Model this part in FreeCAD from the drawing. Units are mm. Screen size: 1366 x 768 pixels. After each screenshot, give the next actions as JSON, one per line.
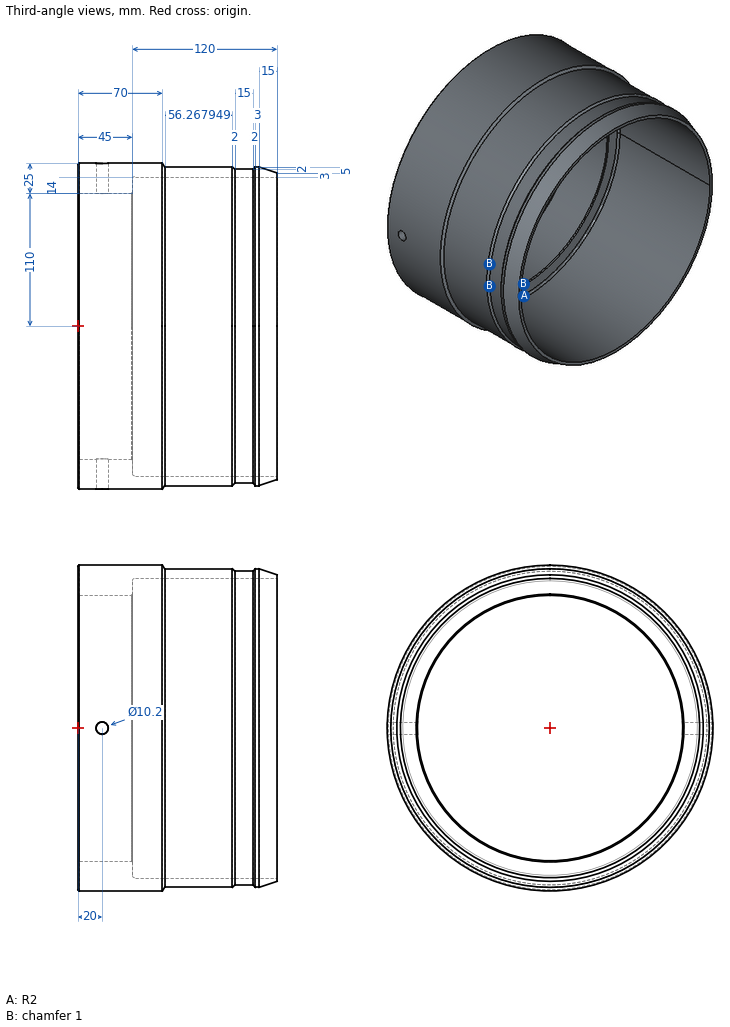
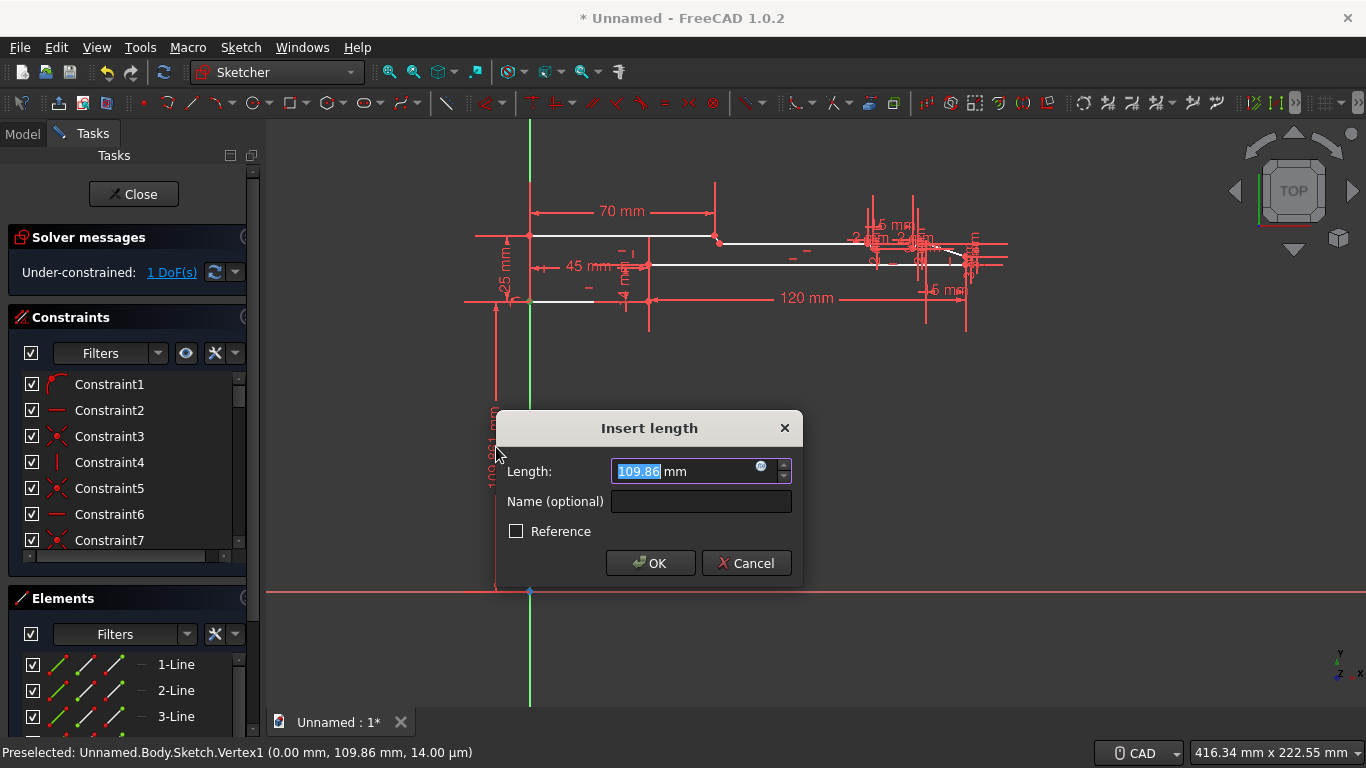
{"action": "type", "text": "110"}
{"action": "key", "text": "Return"}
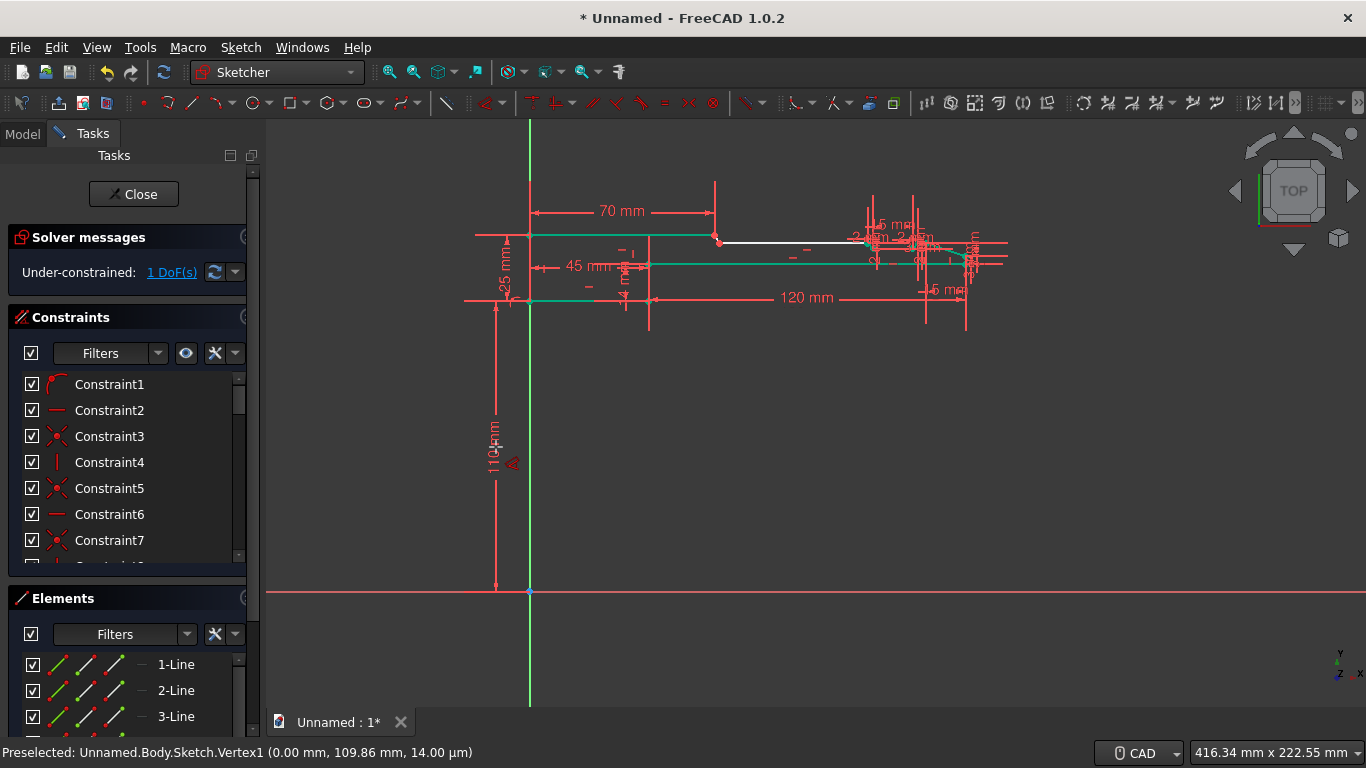
{"action": "left_click", "coordinate": [823, 243]}
{"action": "left_click", "coordinate": [794, 209]}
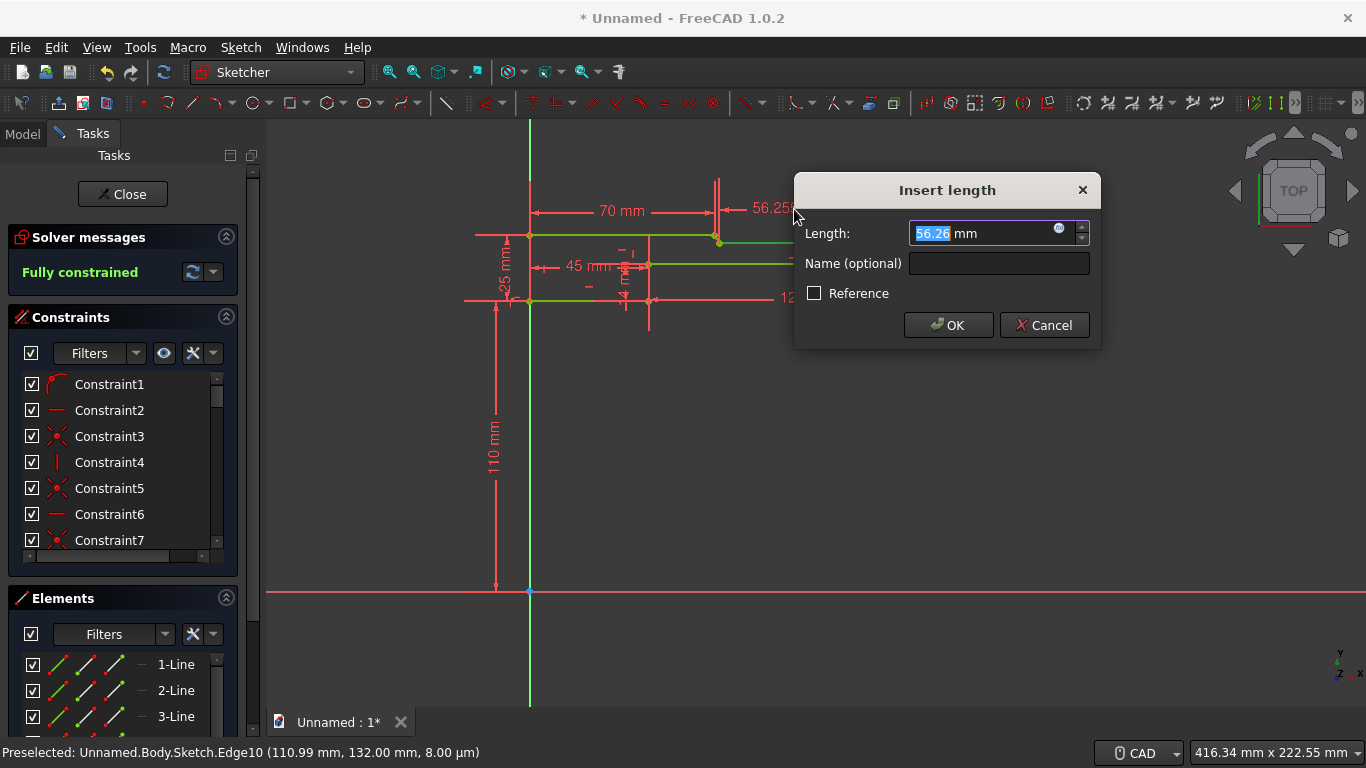
{"action": "type", "text": "56.267949"}
{"action": "key", "text": "Return"}
{"action": "key", "text": "Escape"}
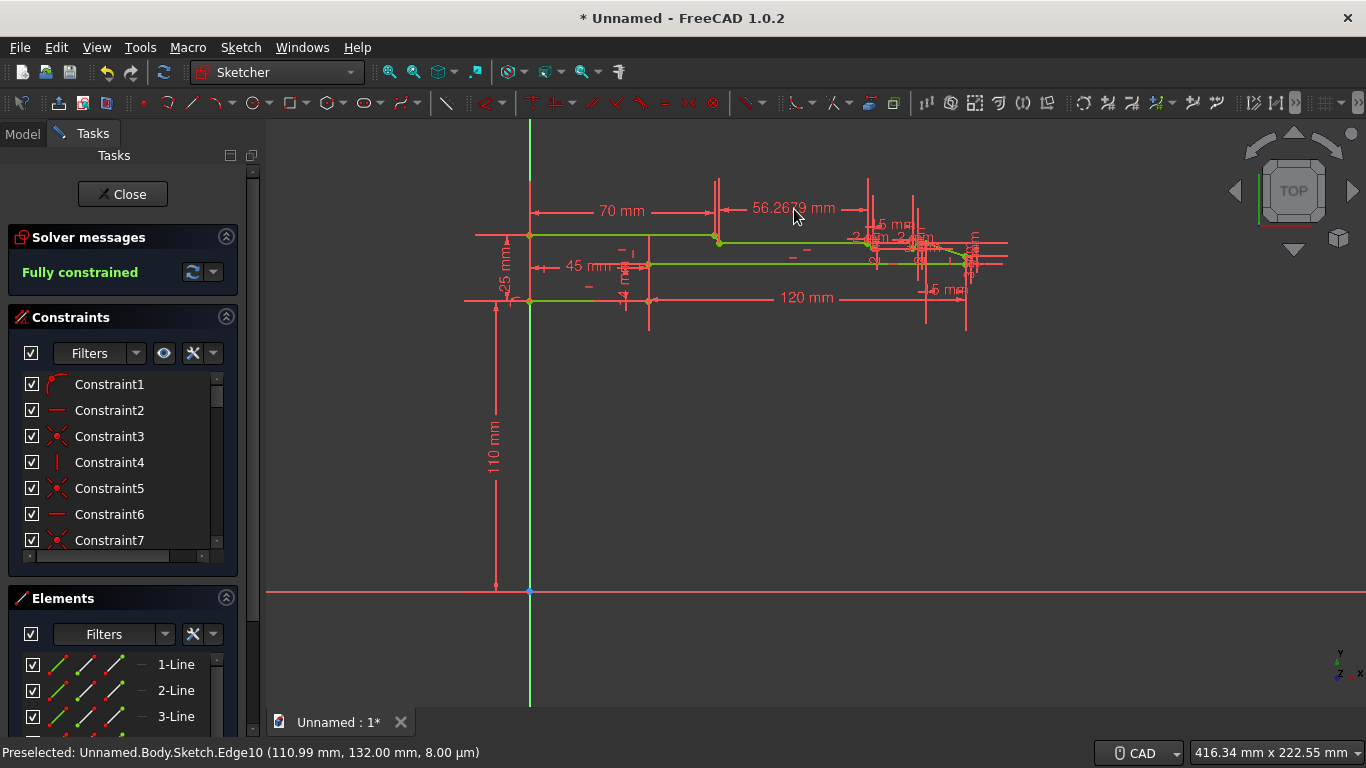
{"action": "left_click", "coordinate": [123, 194]}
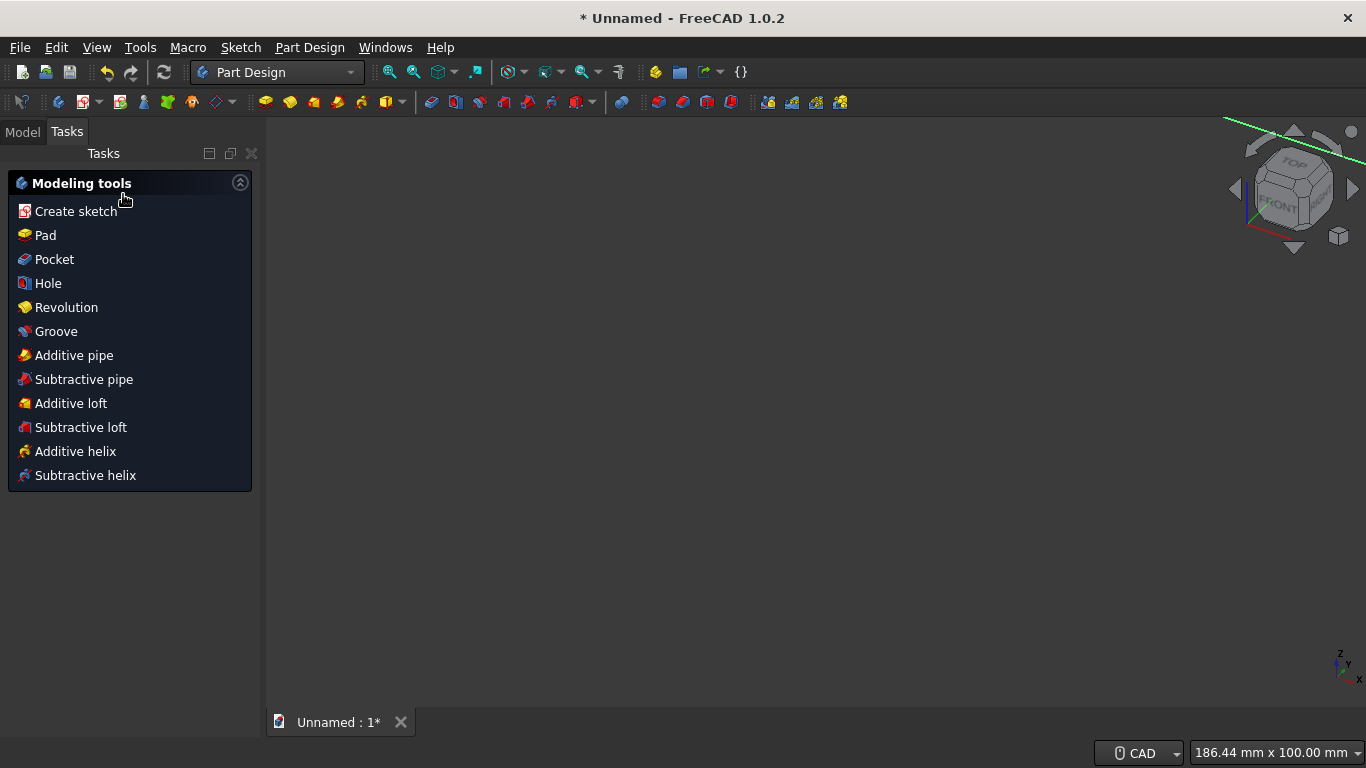
{"action": "left_click", "coordinate": [290, 102]}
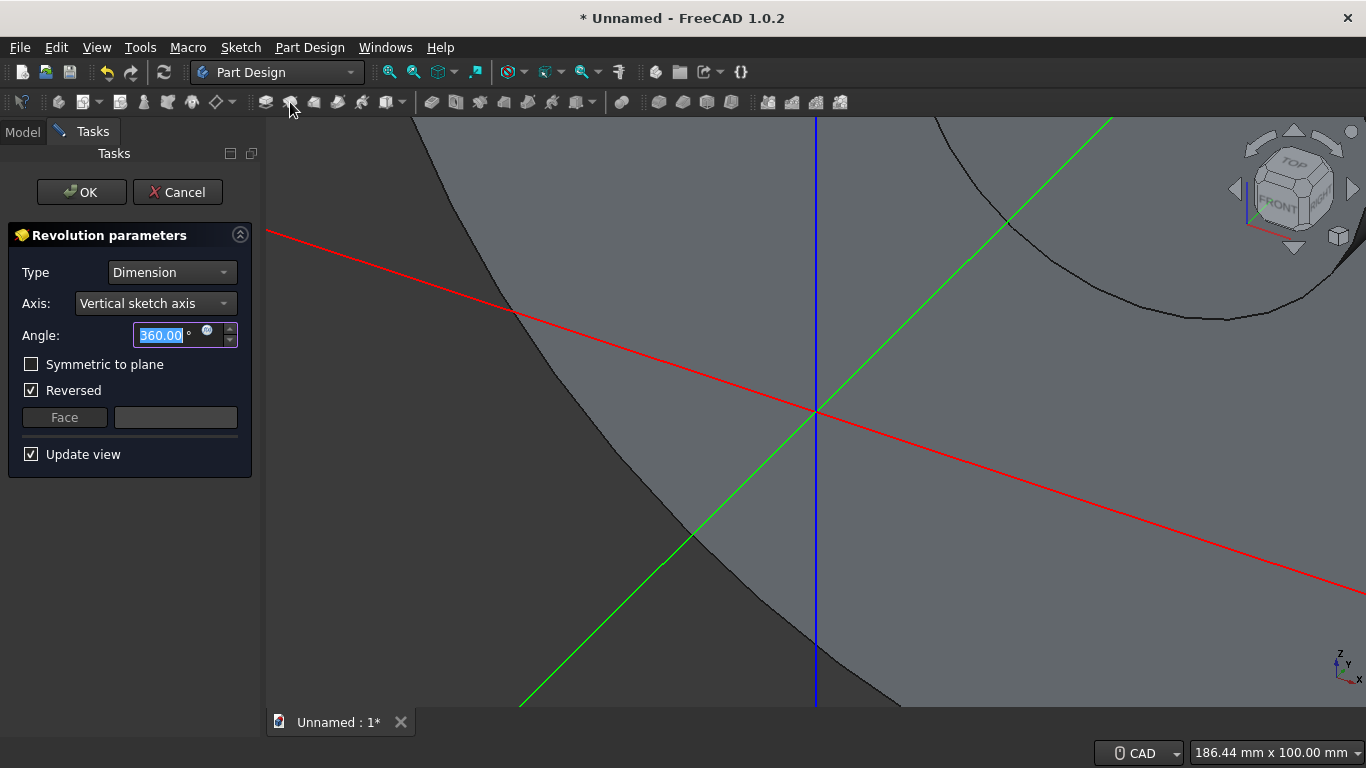
{"action": "left_click", "coordinate": [156, 304]}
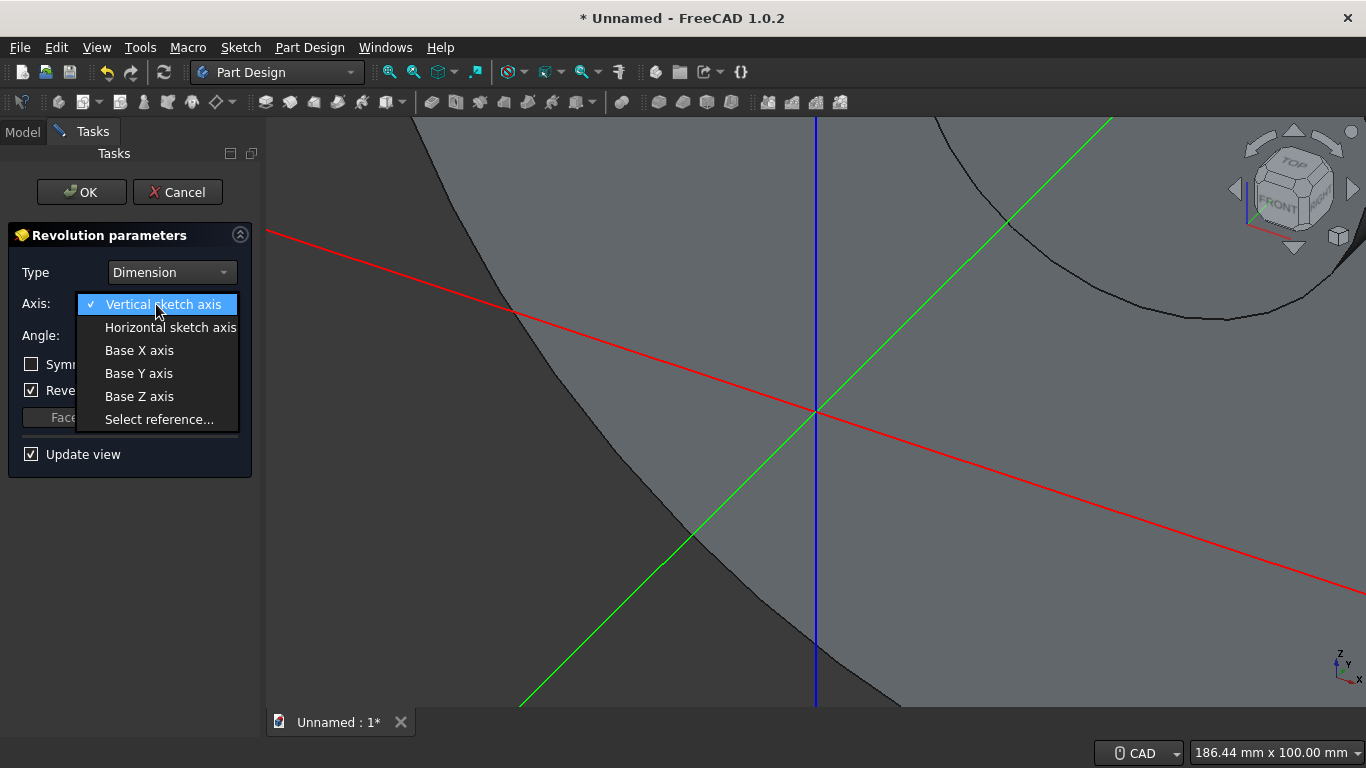
{"action": "left_click", "coordinate": [156, 328]}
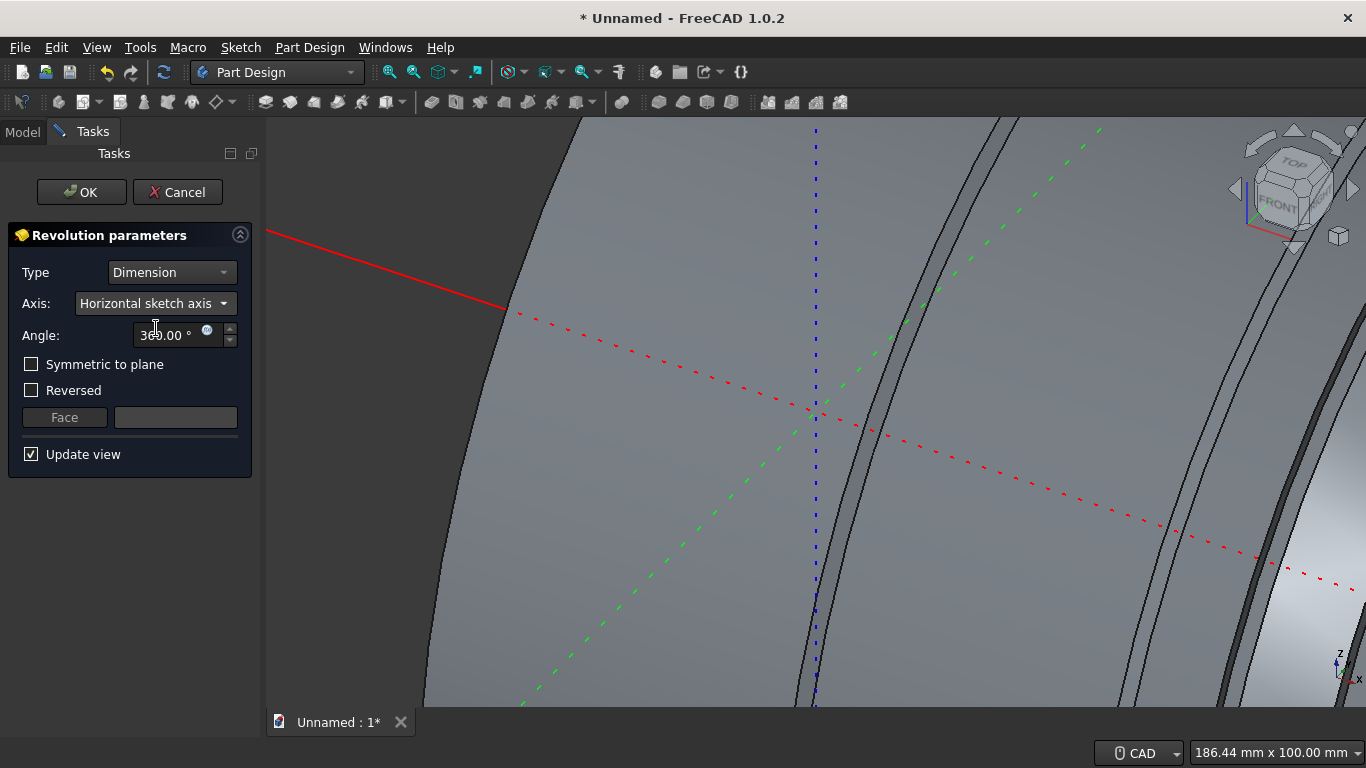
{"action": "left_click", "coordinate": [82, 192]}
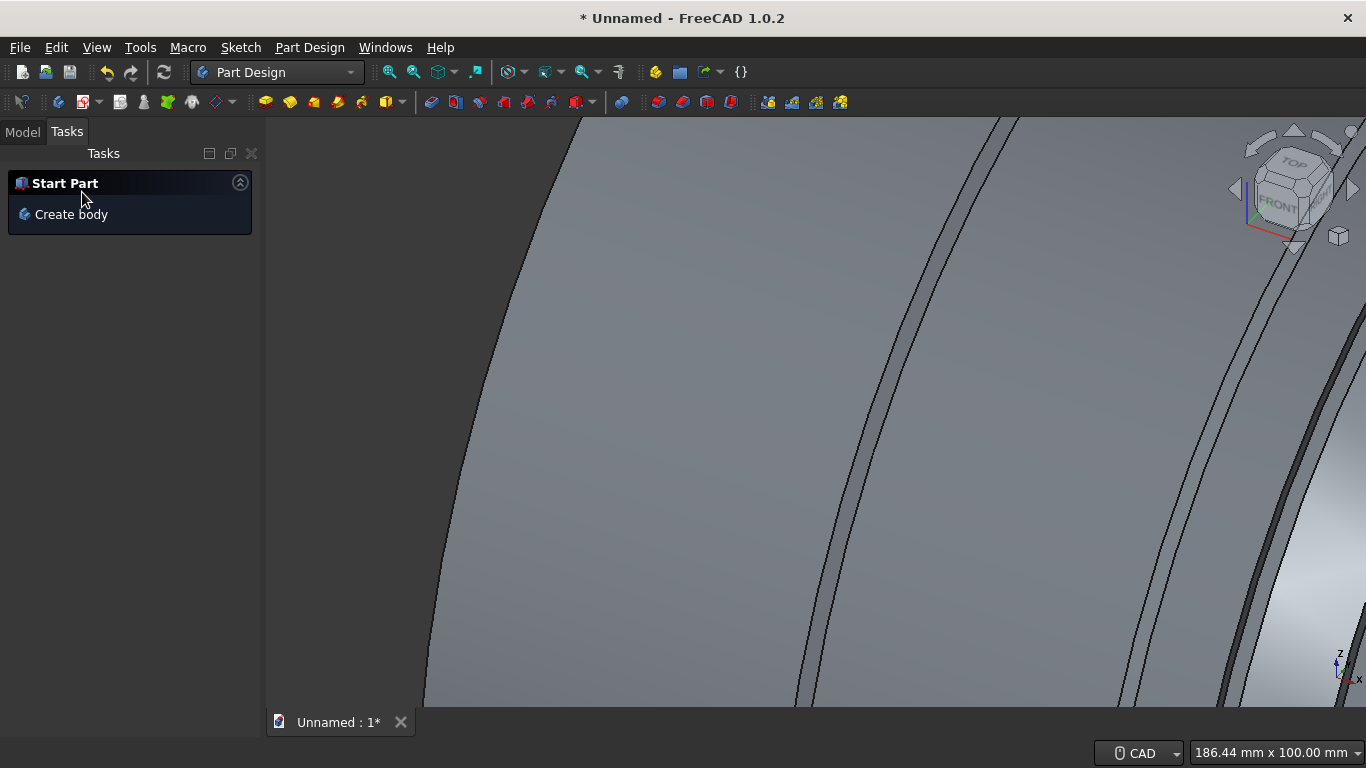
{"action": "left_click", "coordinate": [390, 72]}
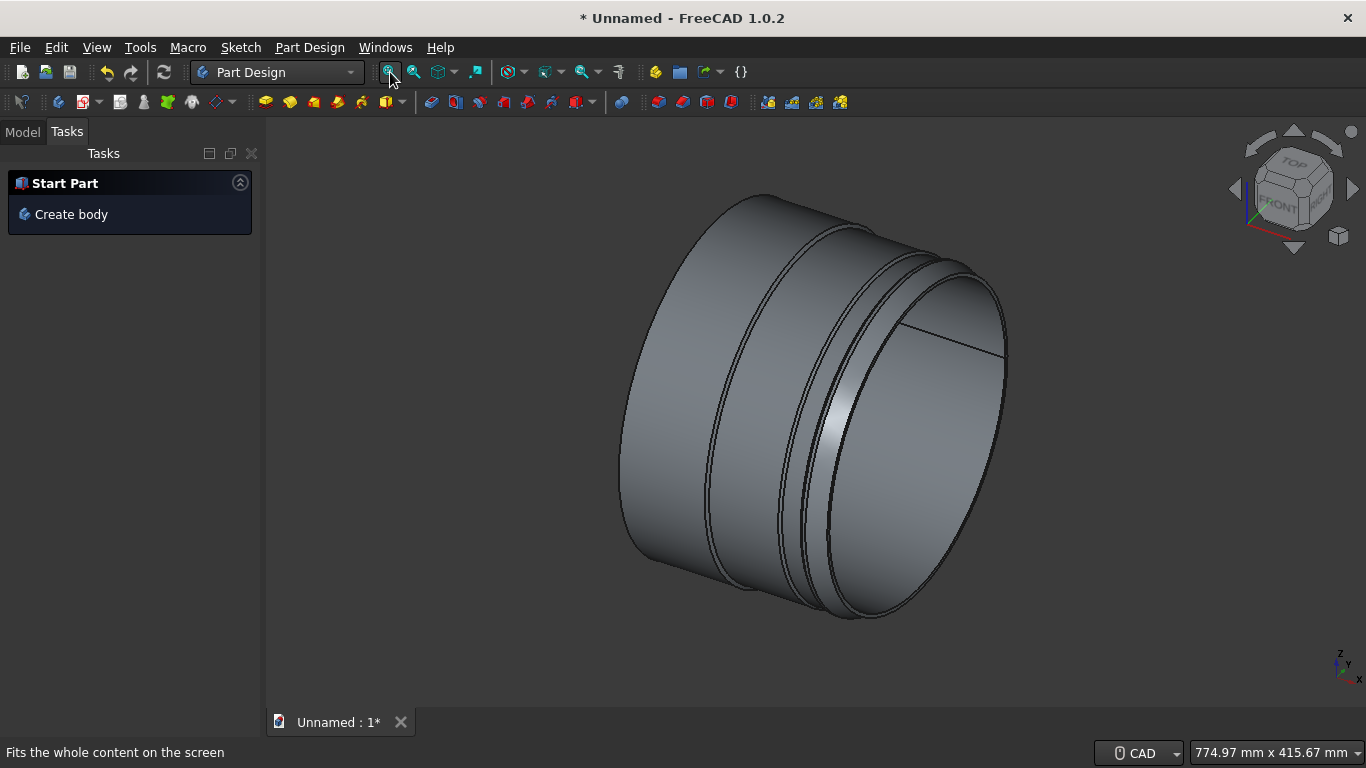
{"action": "key", "text": "0"}